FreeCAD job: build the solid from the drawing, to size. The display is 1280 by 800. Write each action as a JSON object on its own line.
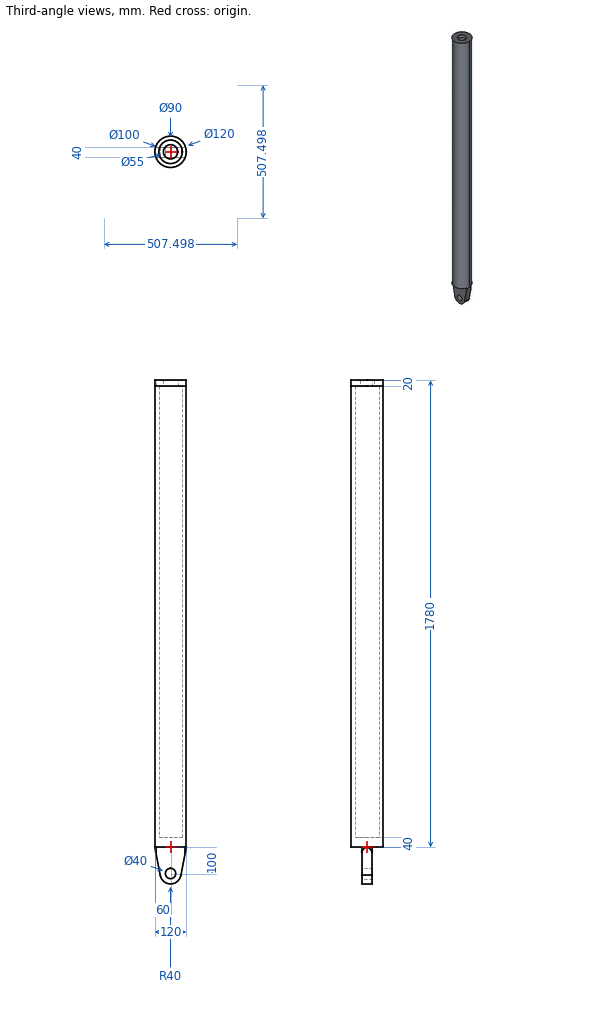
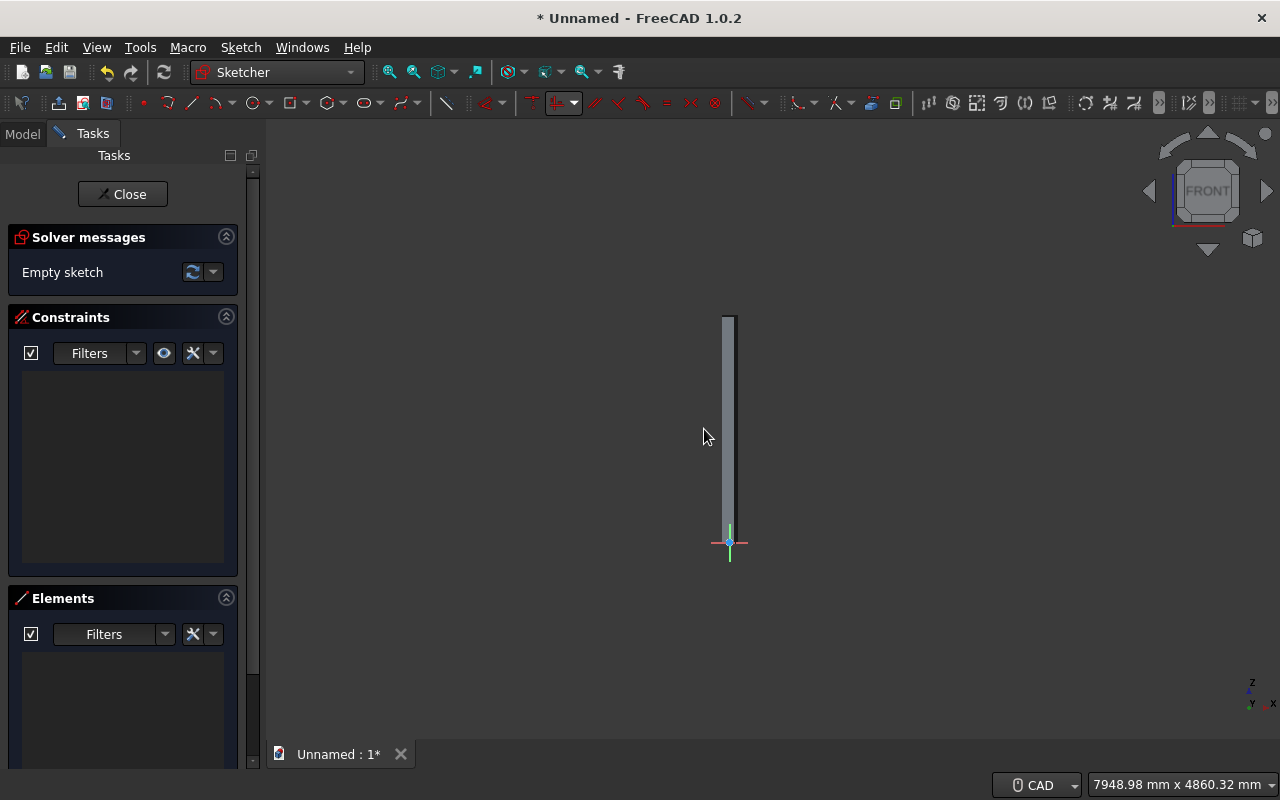
{"action": "scroll", "coordinate": [731, 558], "scroll_direction": "up", "scroll_amount": 15}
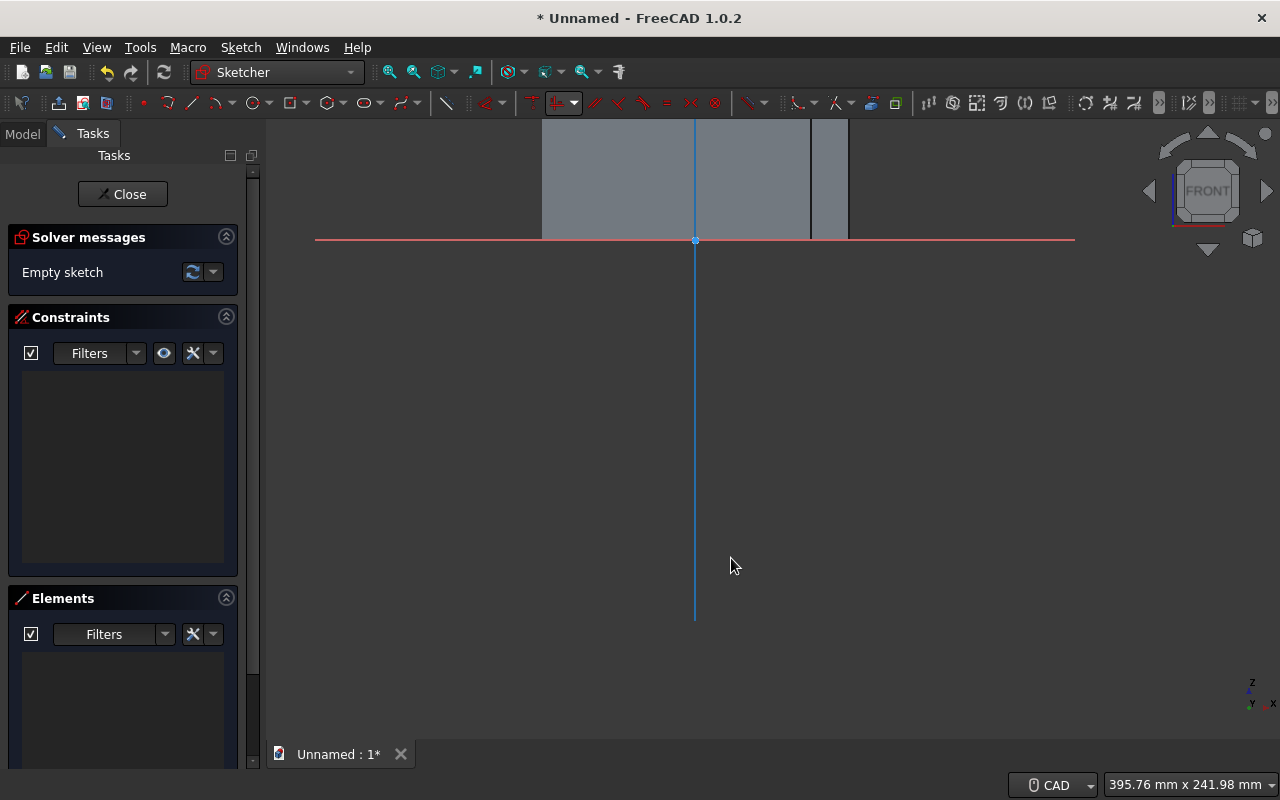
{"action": "left_click", "coordinate": [168, 104]}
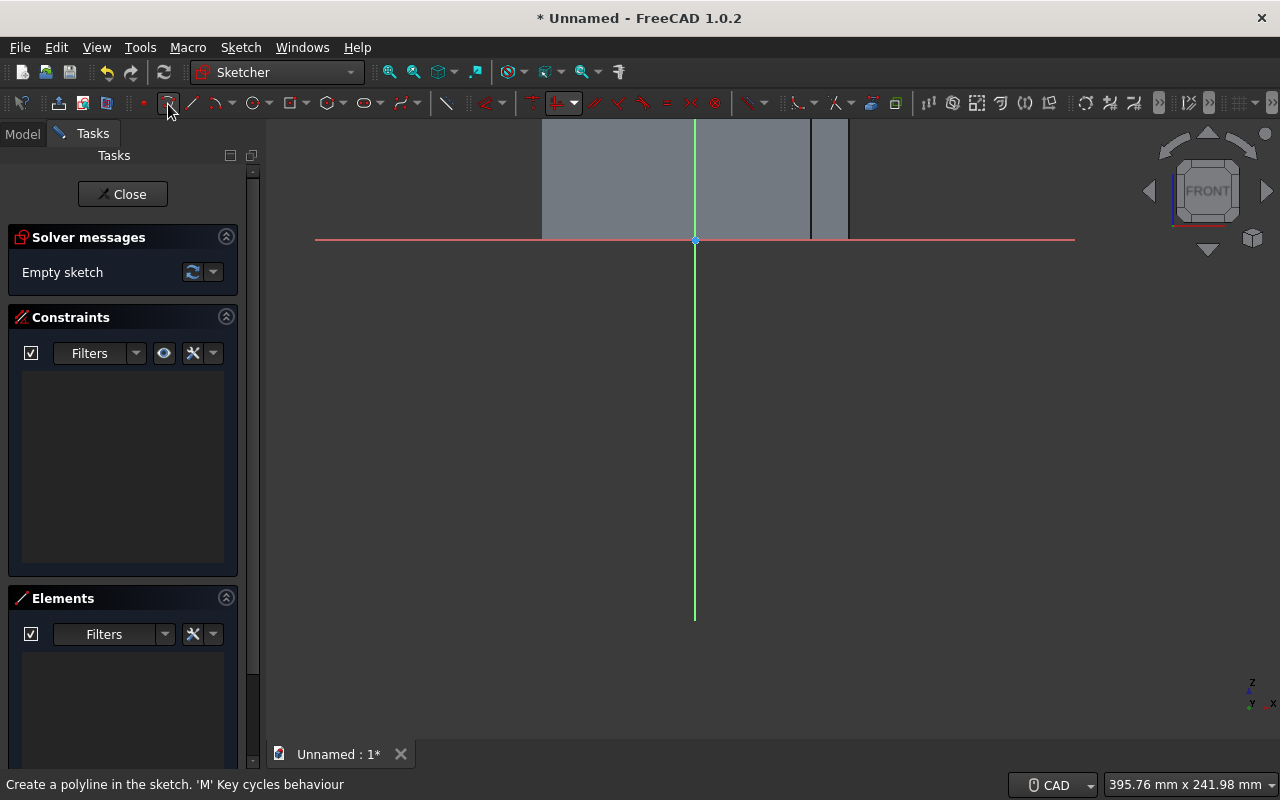
{"action": "left_click", "coordinate": [595, 516]}
{"action": "left_click", "coordinate": [542, 240]}
{"action": "left_click", "coordinate": [849, 249]}
{"action": "left_click", "coordinate": [796, 516]}
{"action": "right_click", "coordinate": [796, 516]}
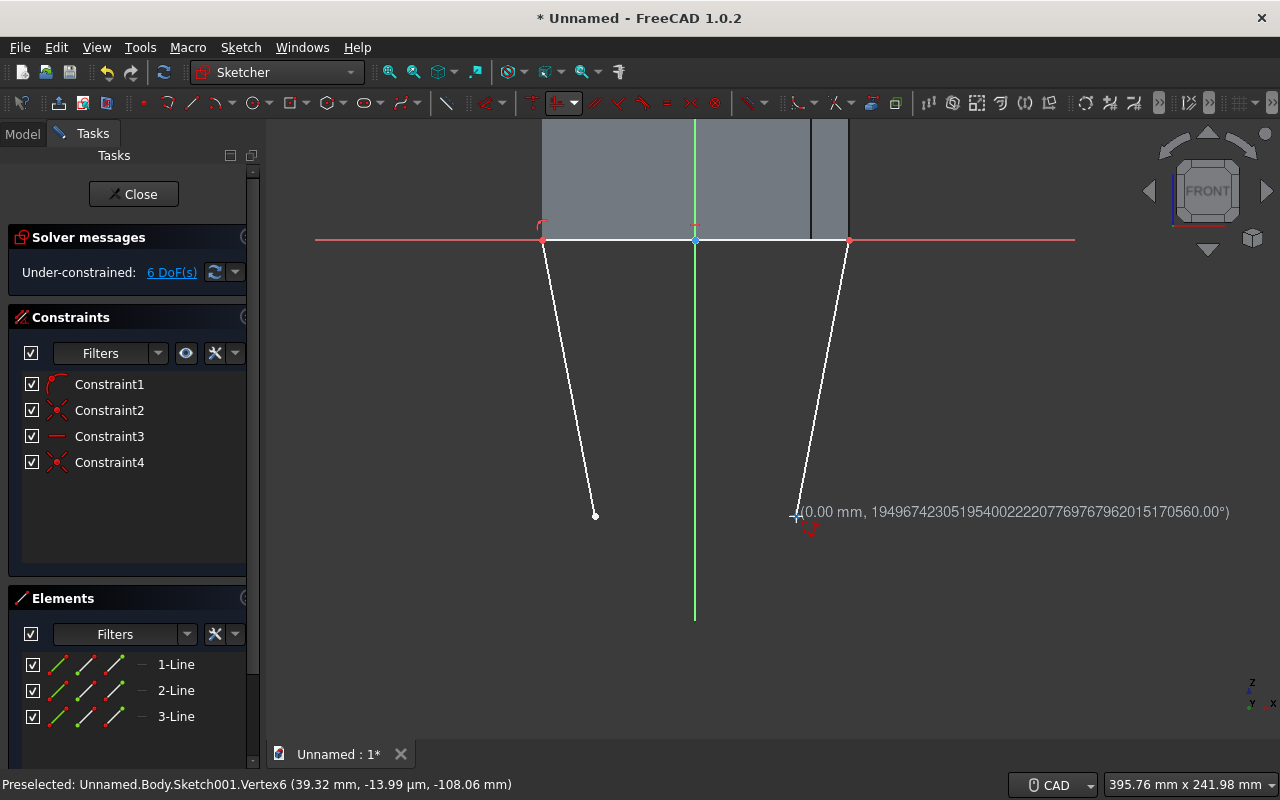
{"action": "key", "text": "g 3 a"}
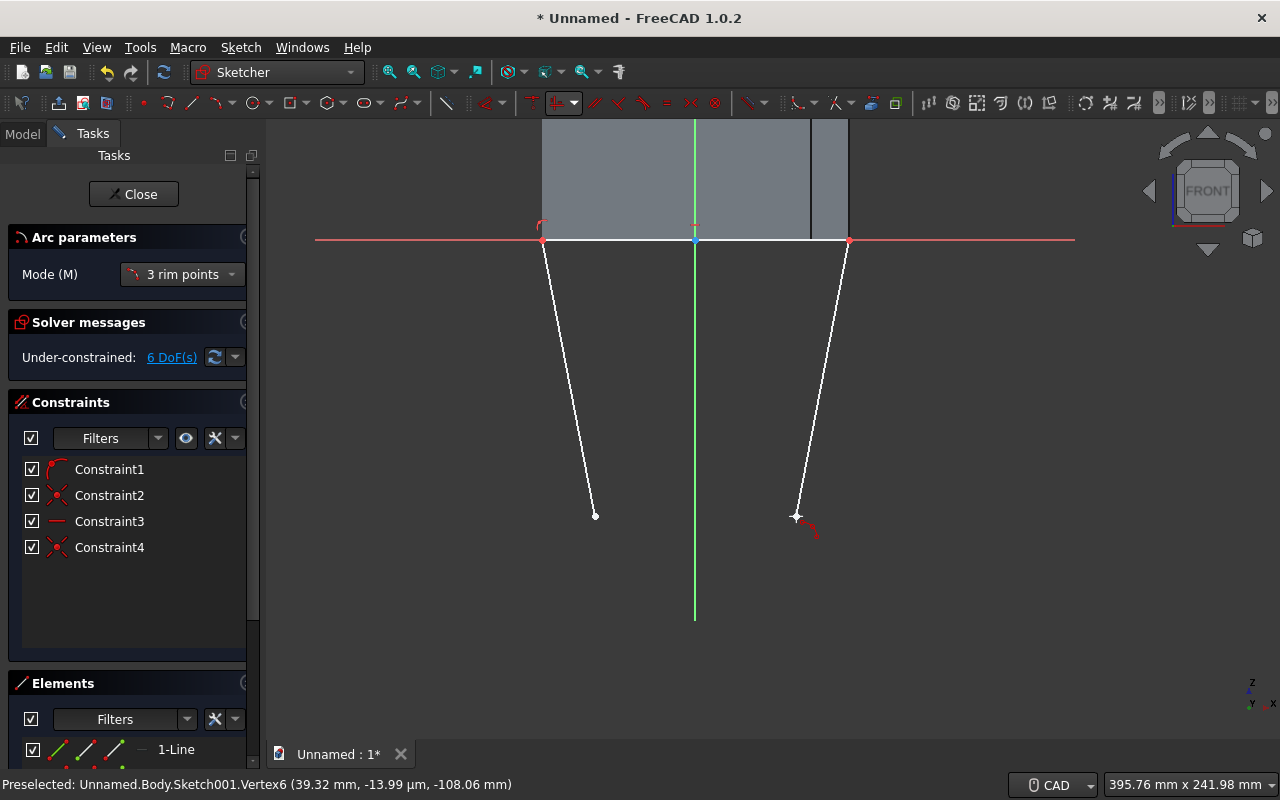
{"action": "left_click", "coordinate": [796, 517]}
{"action": "left_click", "coordinate": [595, 517]}
{"action": "left_click", "coordinate": [667, 595]}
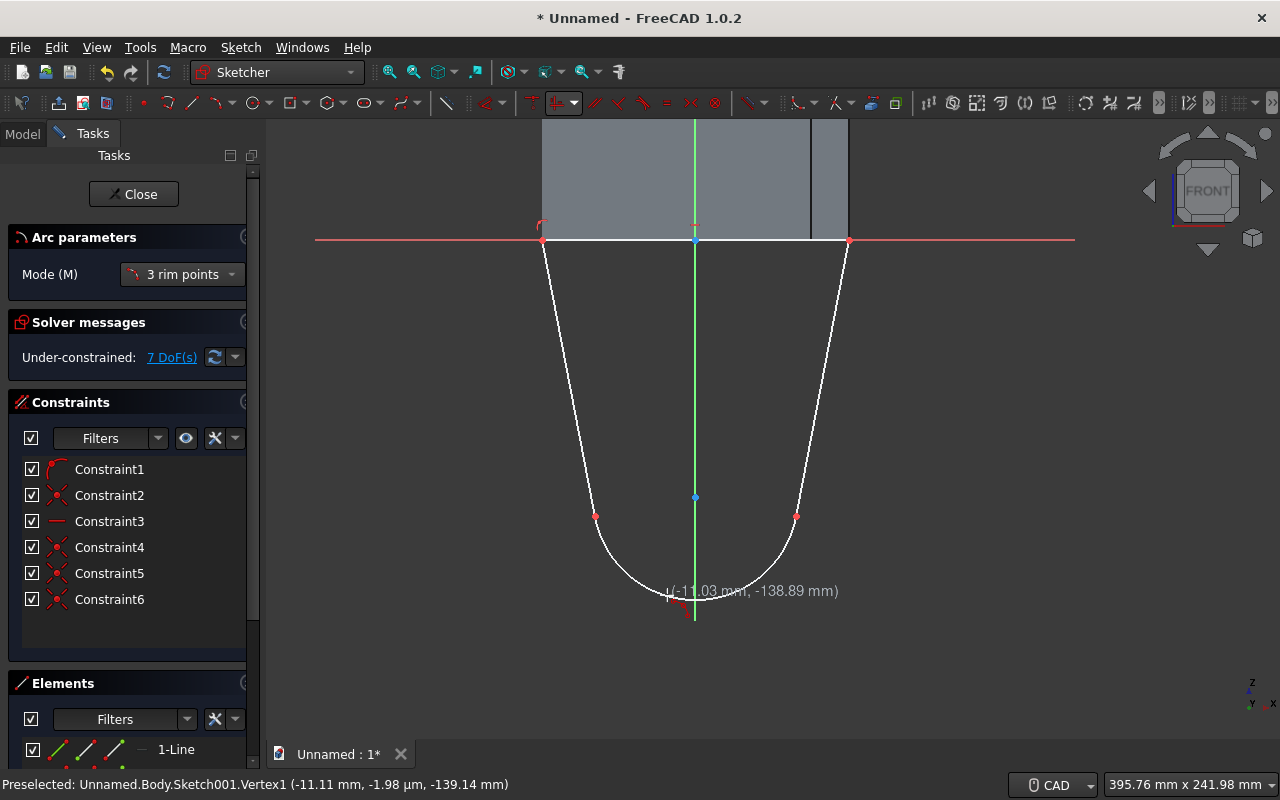
{"action": "left_click", "coordinate": [254, 104]}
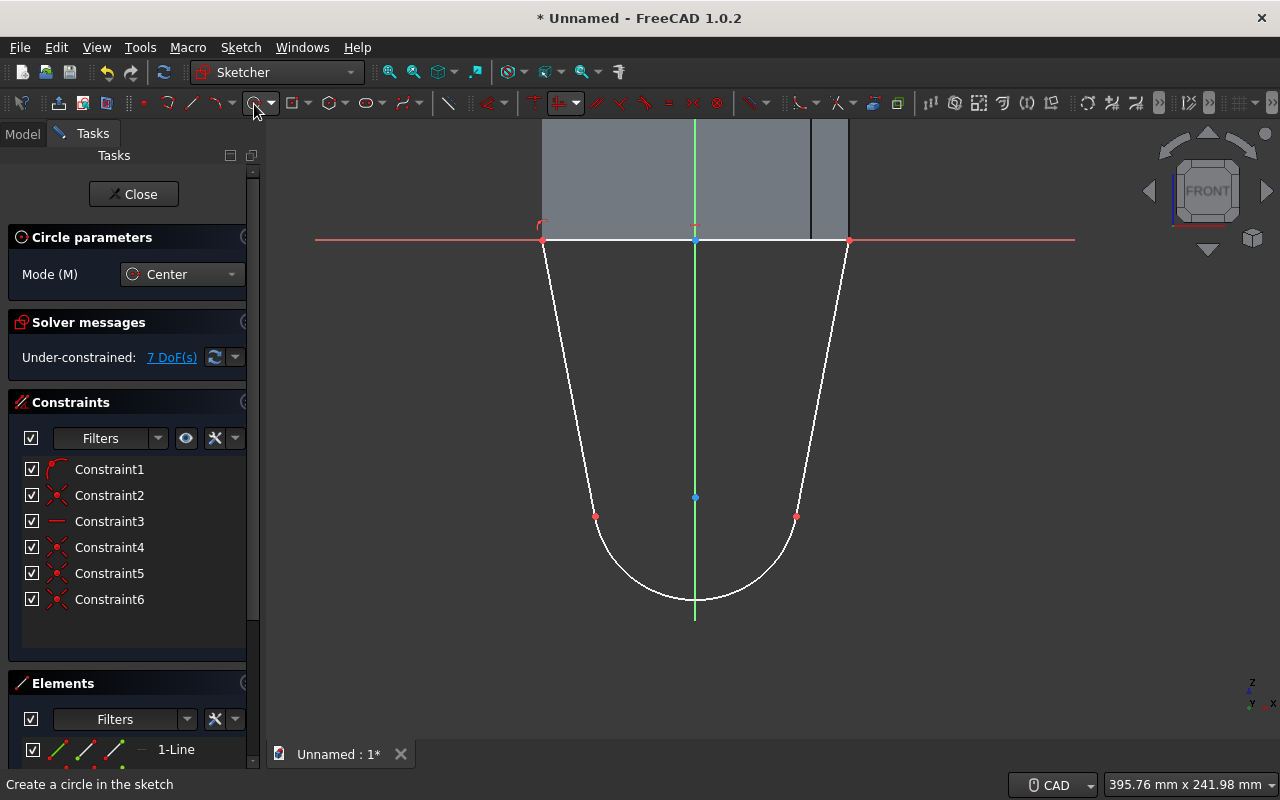
{"action": "left_click", "coordinate": [695, 496]}
{"action": "mouse_move", "coordinate": [731, 460]}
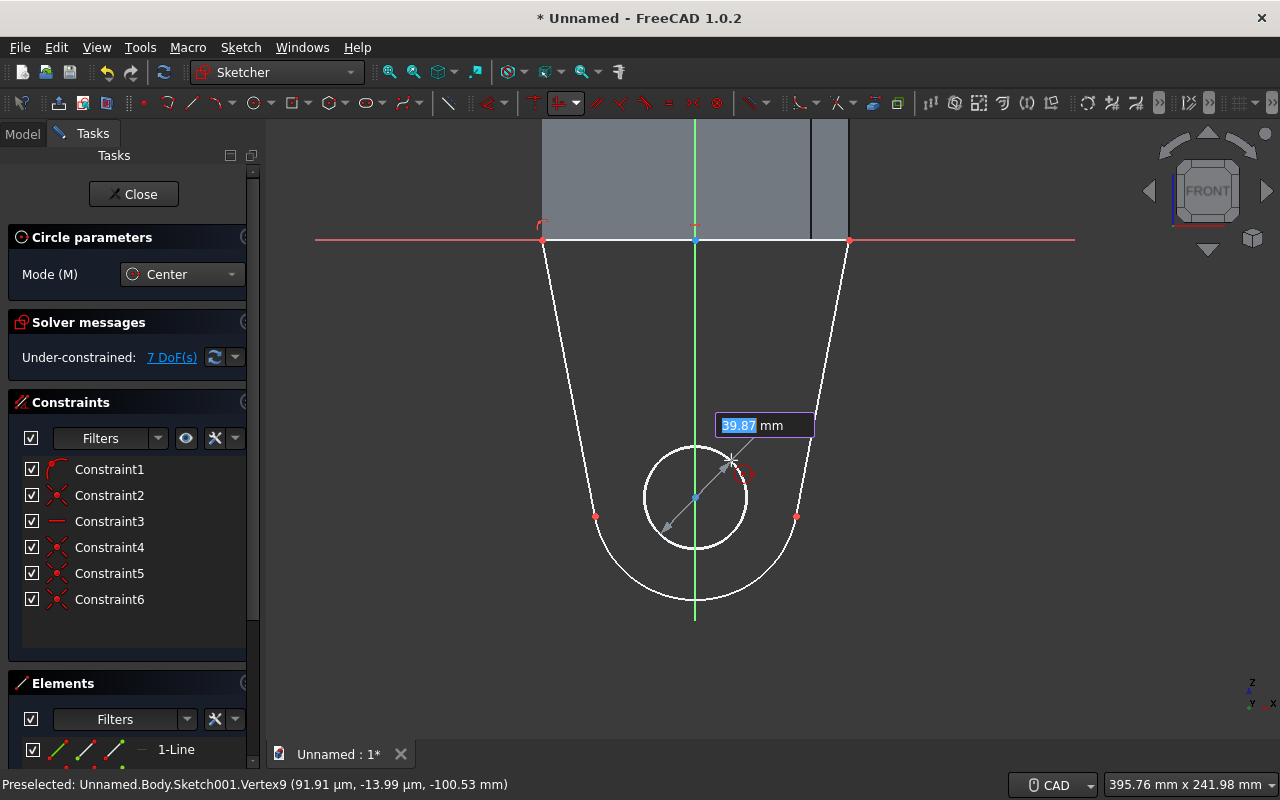
{"action": "type", "text": "40"}
{"action": "key", "text": "Return"}
{"action": "key", "text": "Escape"}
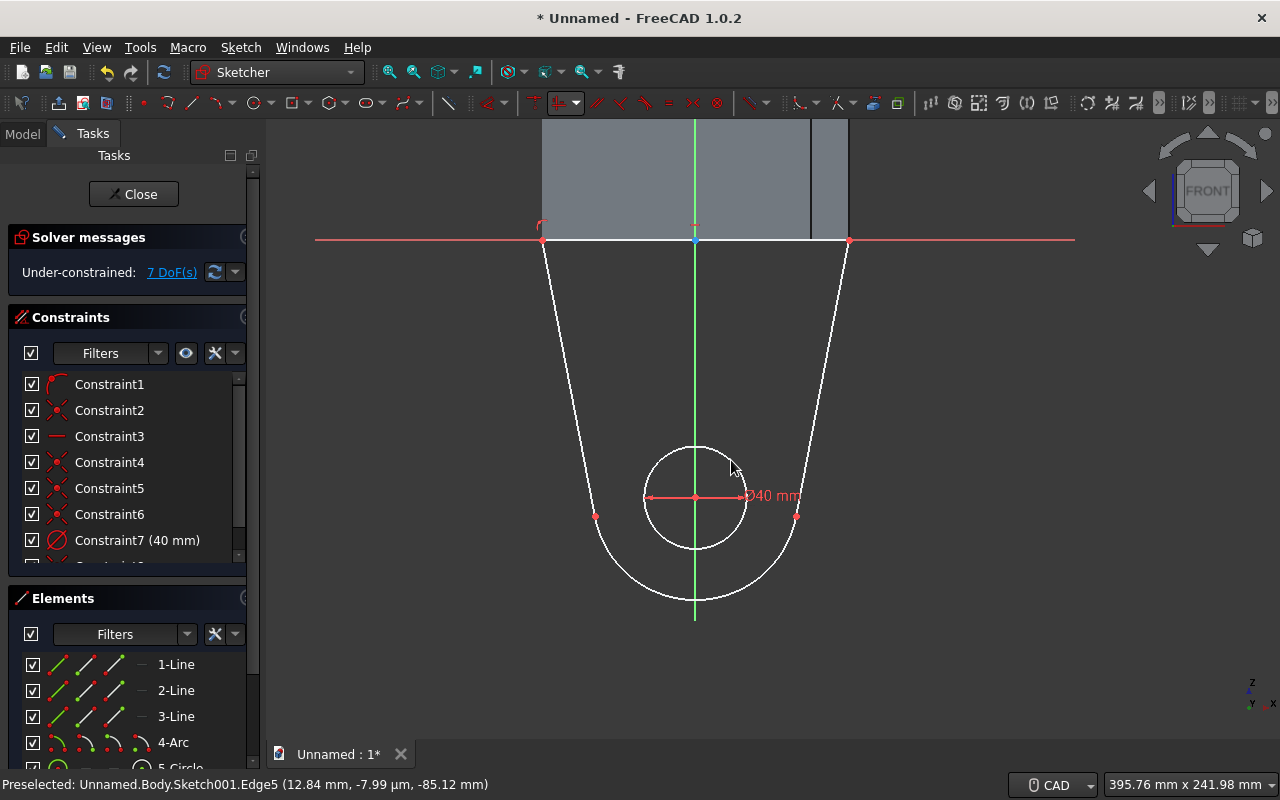
{"action": "left_click", "coordinate": [579, 434]}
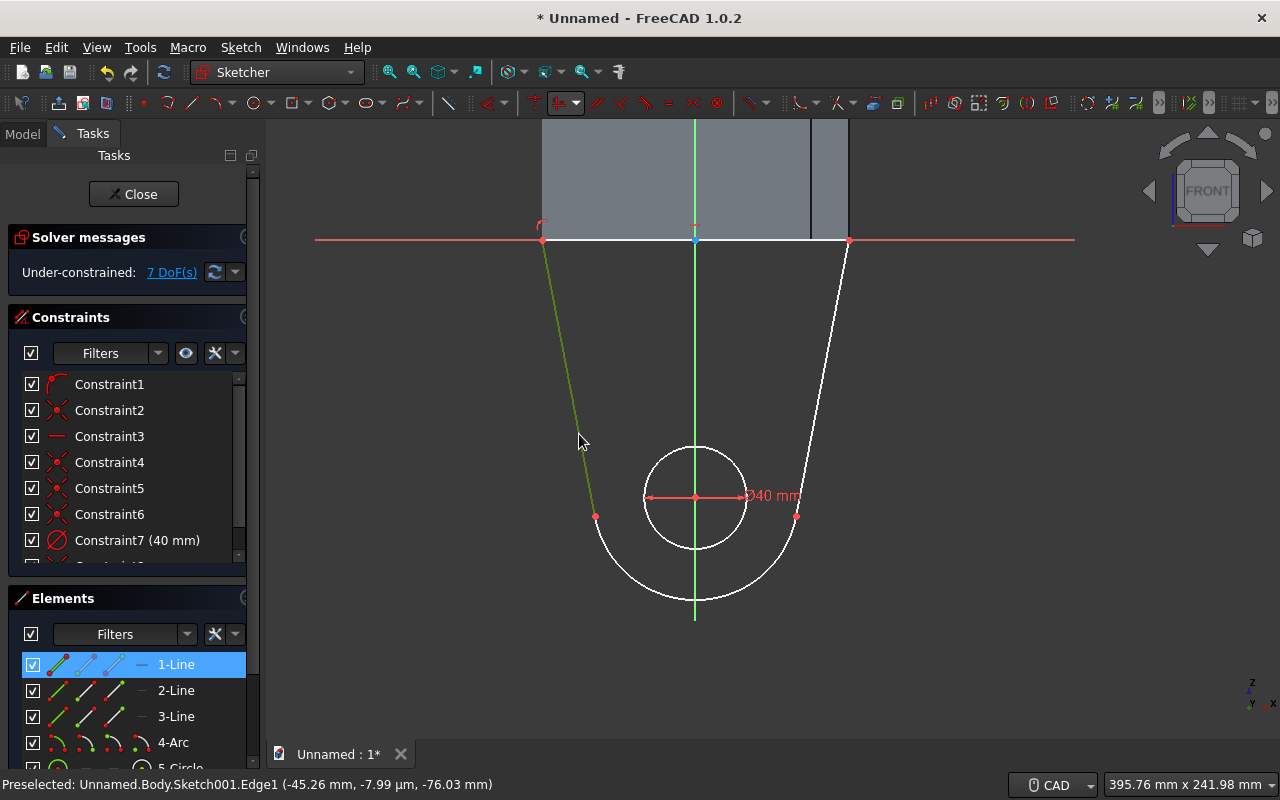
{"action": "left_click", "coordinate": [642, 585]}